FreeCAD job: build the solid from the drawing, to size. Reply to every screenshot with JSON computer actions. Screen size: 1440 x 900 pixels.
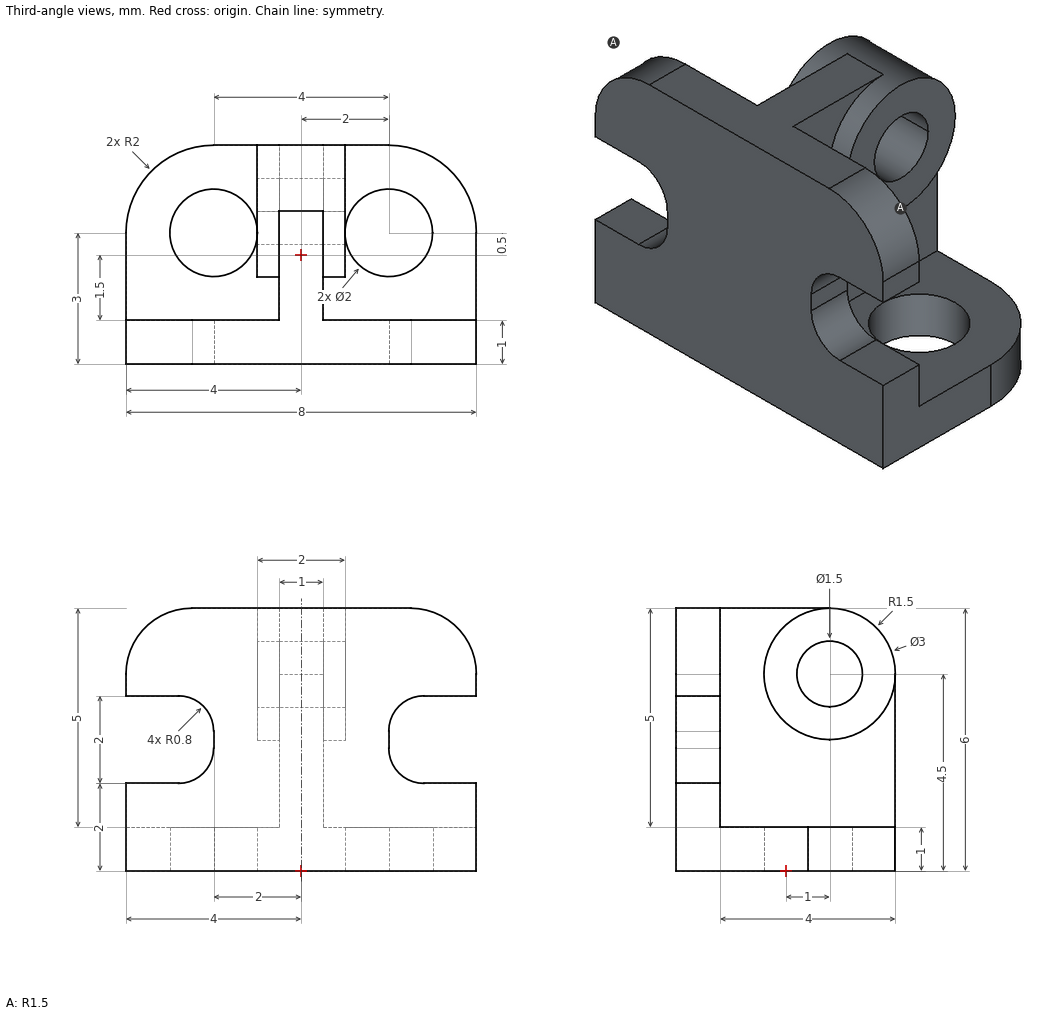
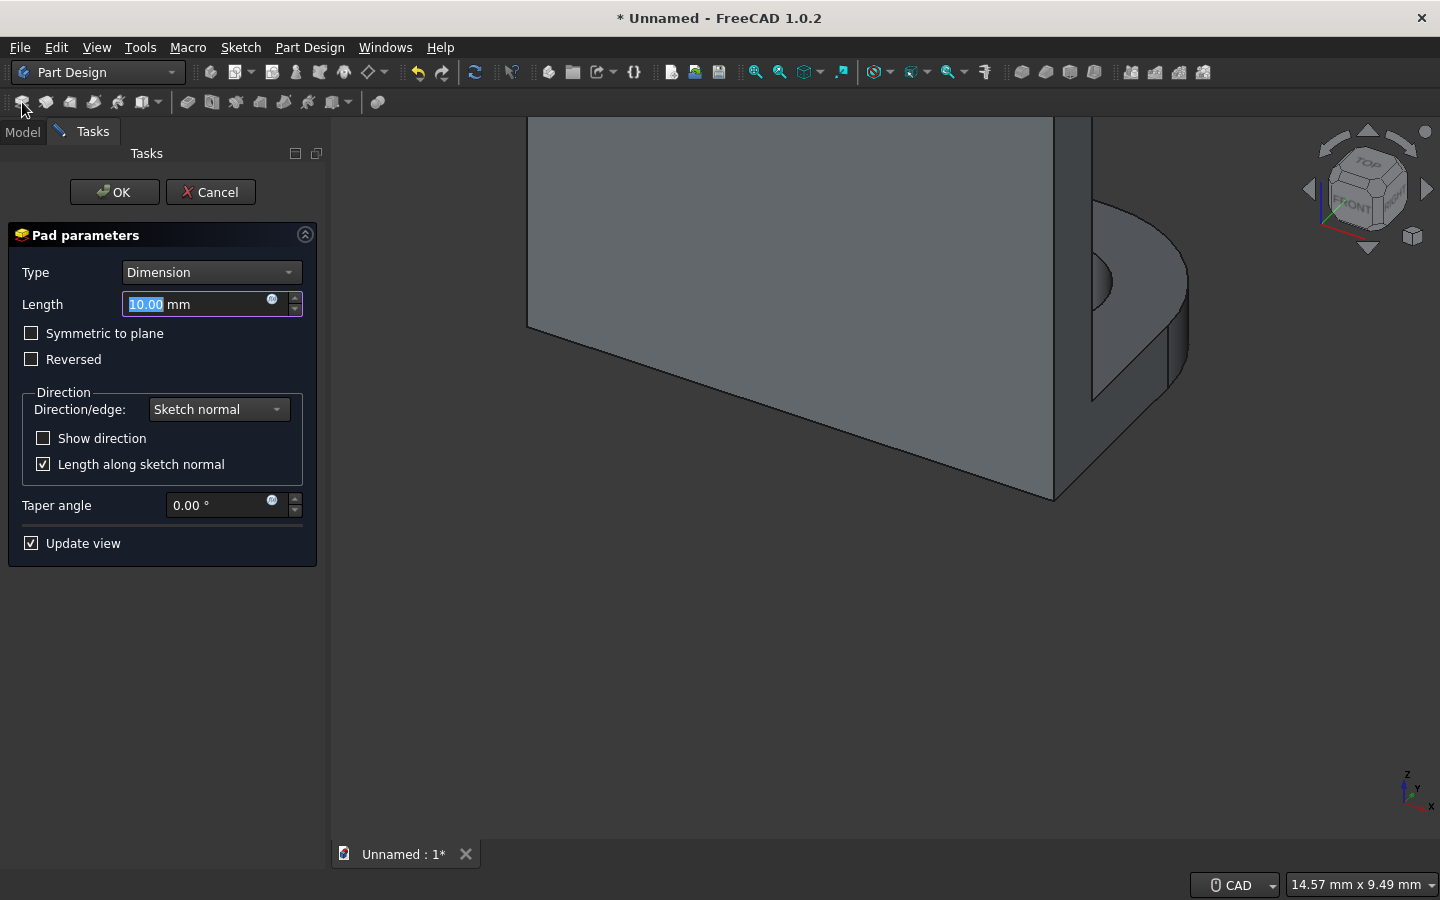
{"action": "type", "text": "5"}
{"action": "key", "text": "Tab"}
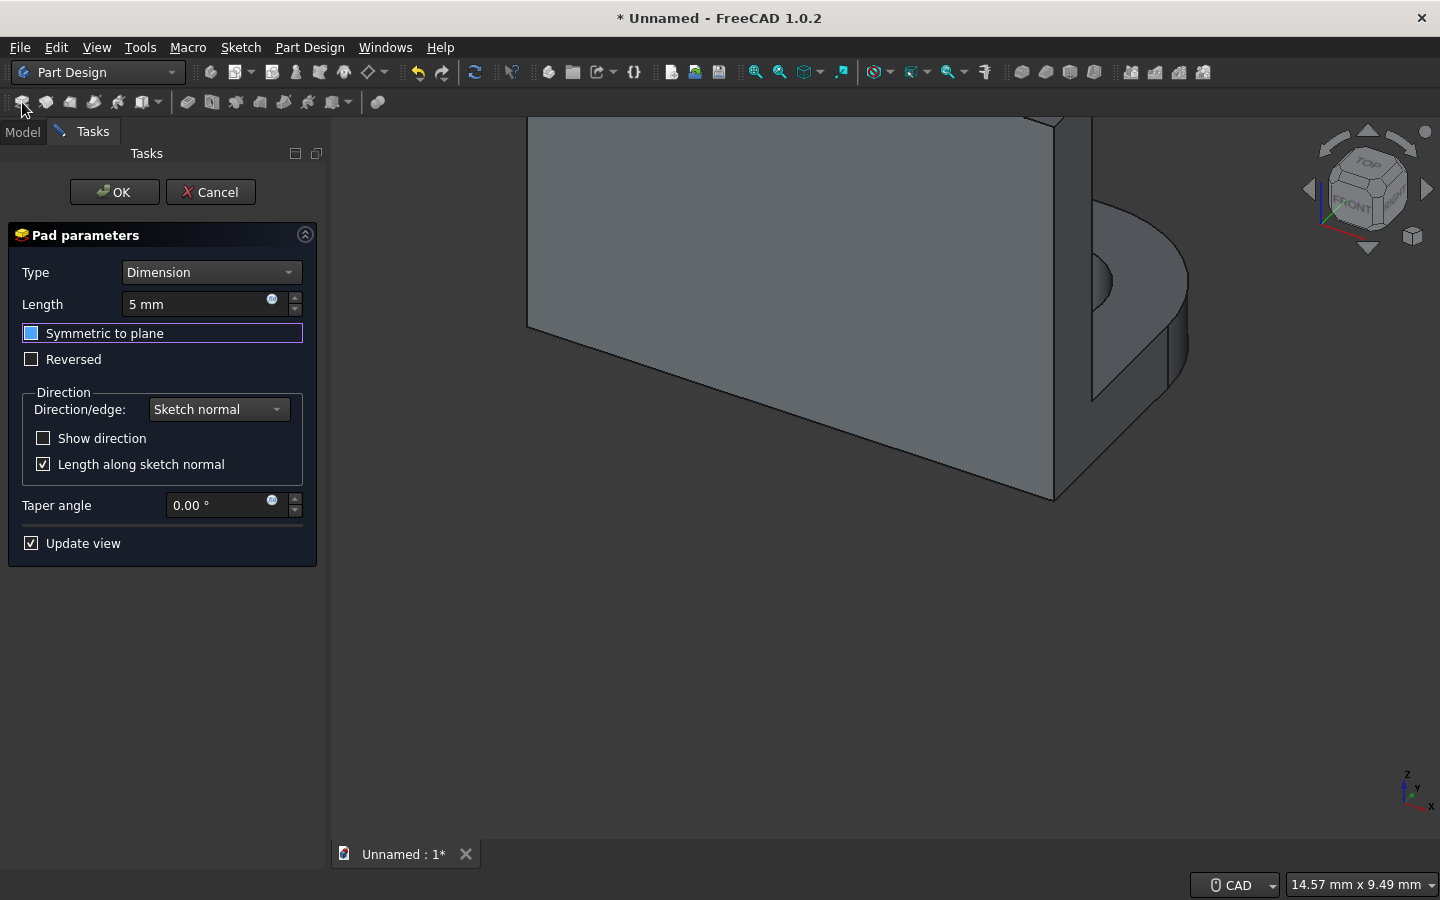
{"action": "left_click", "coordinate": [115, 192]}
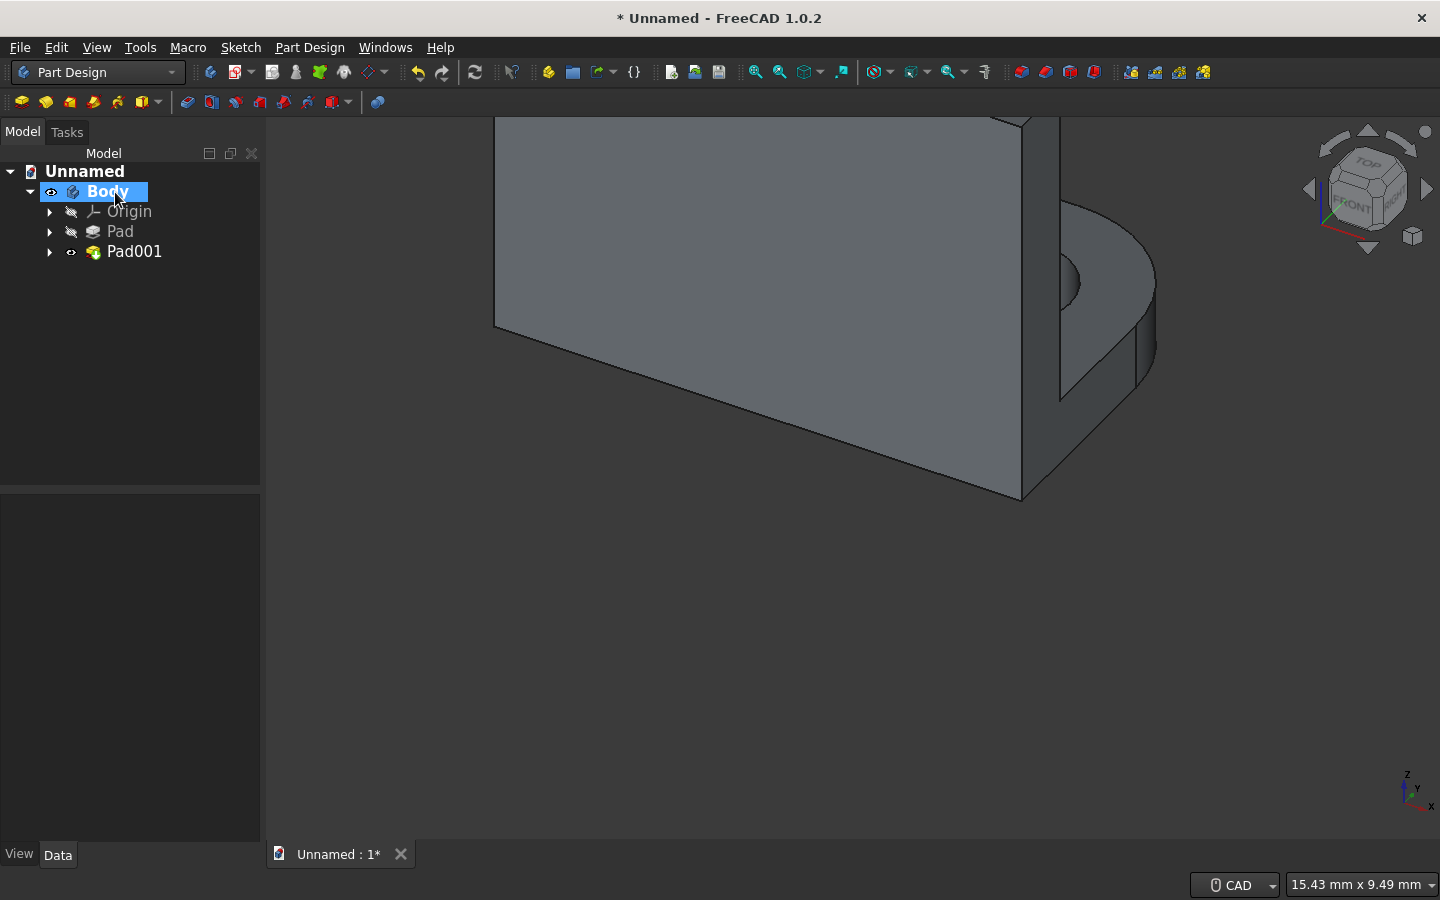
{"action": "left_click", "coordinate": [756, 72]}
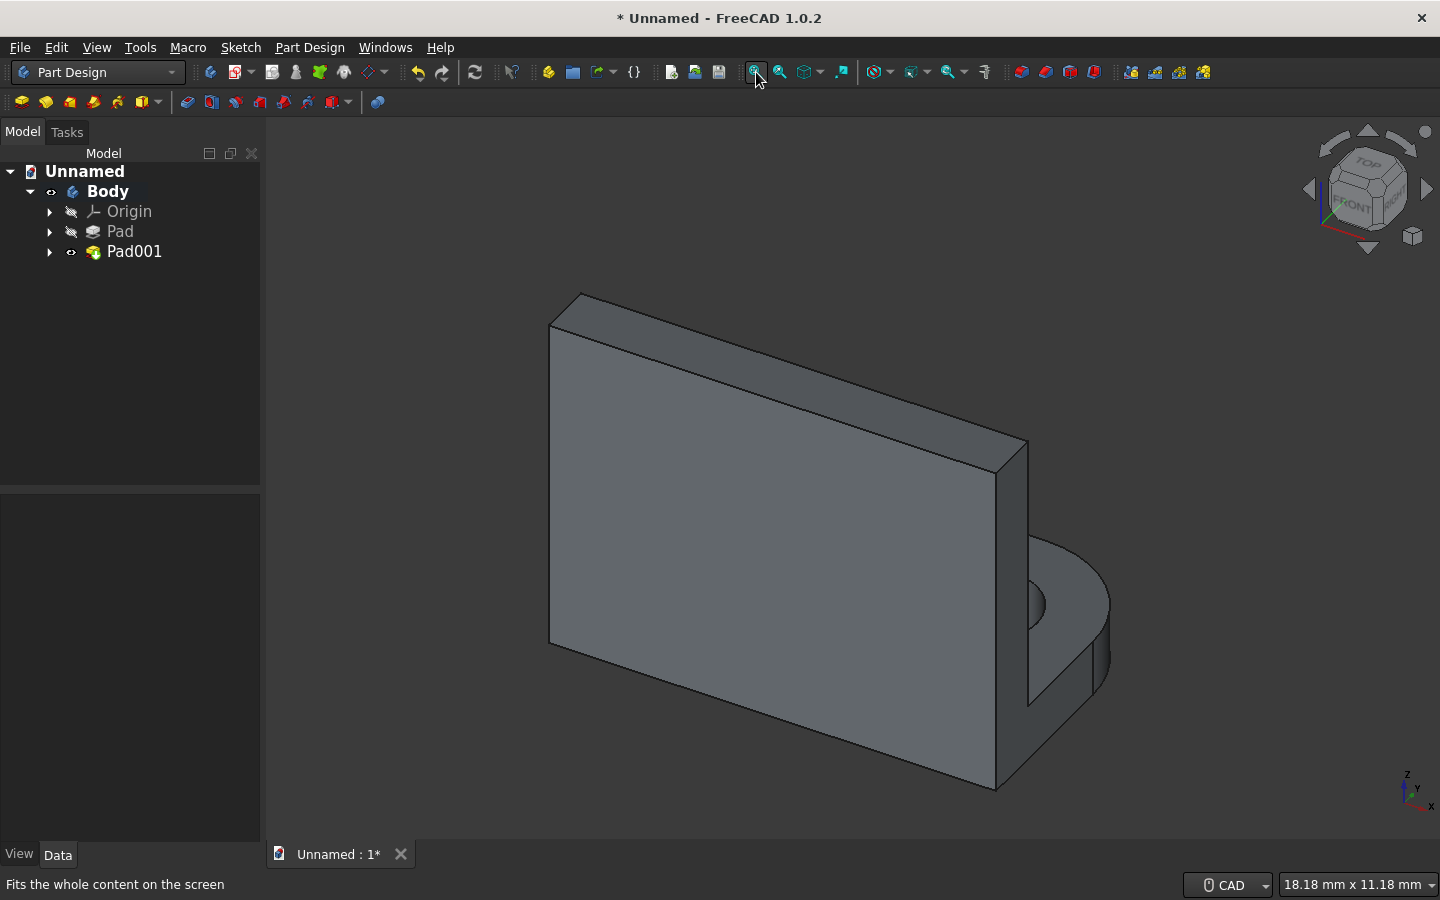
{"action": "key", "text": "4"}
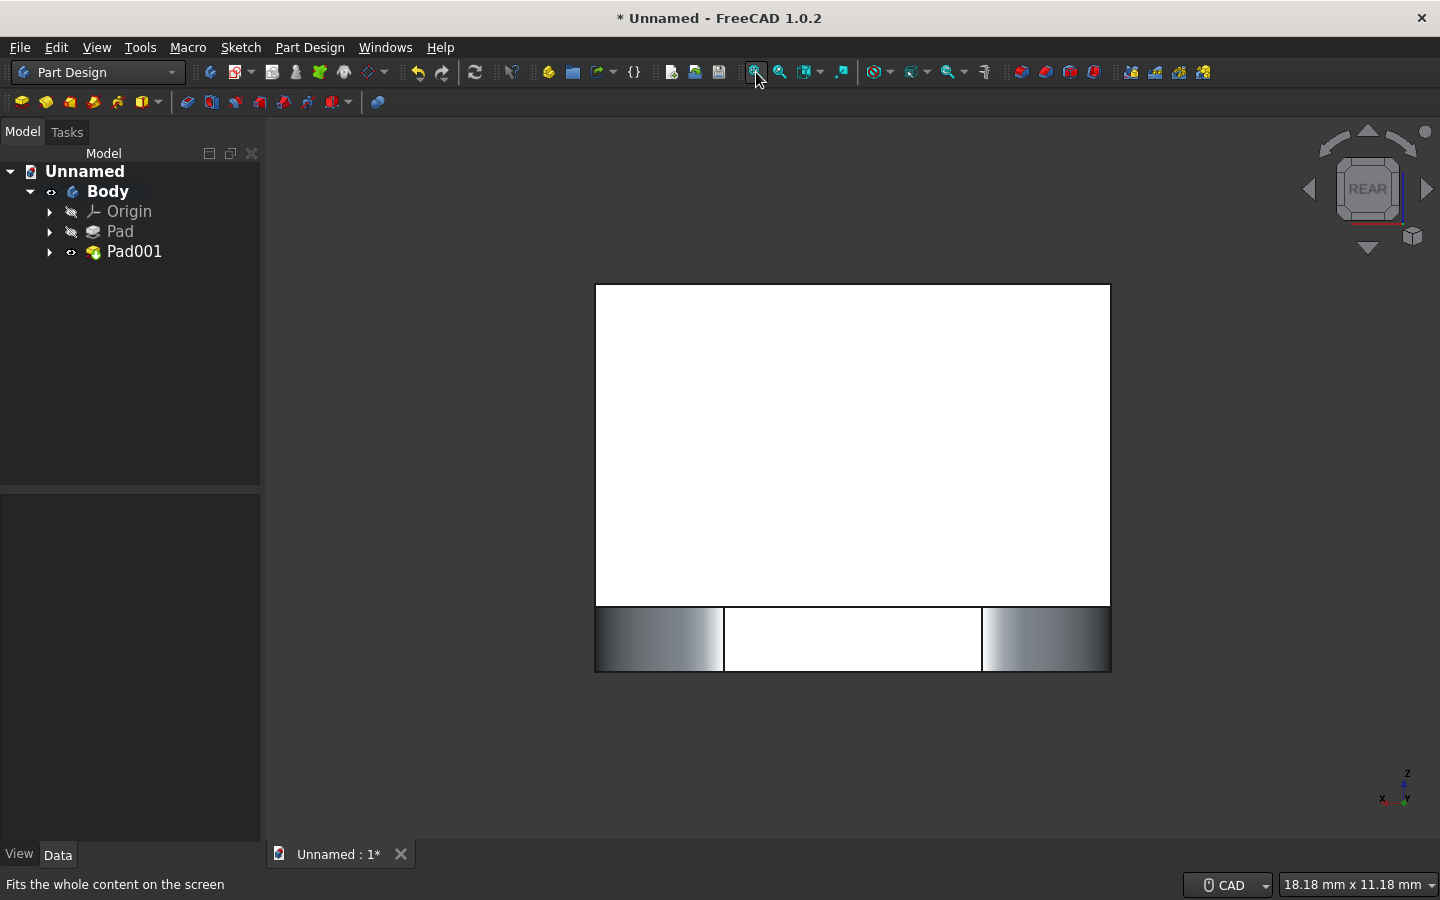
{"action": "left_click", "coordinate": [779, 445]}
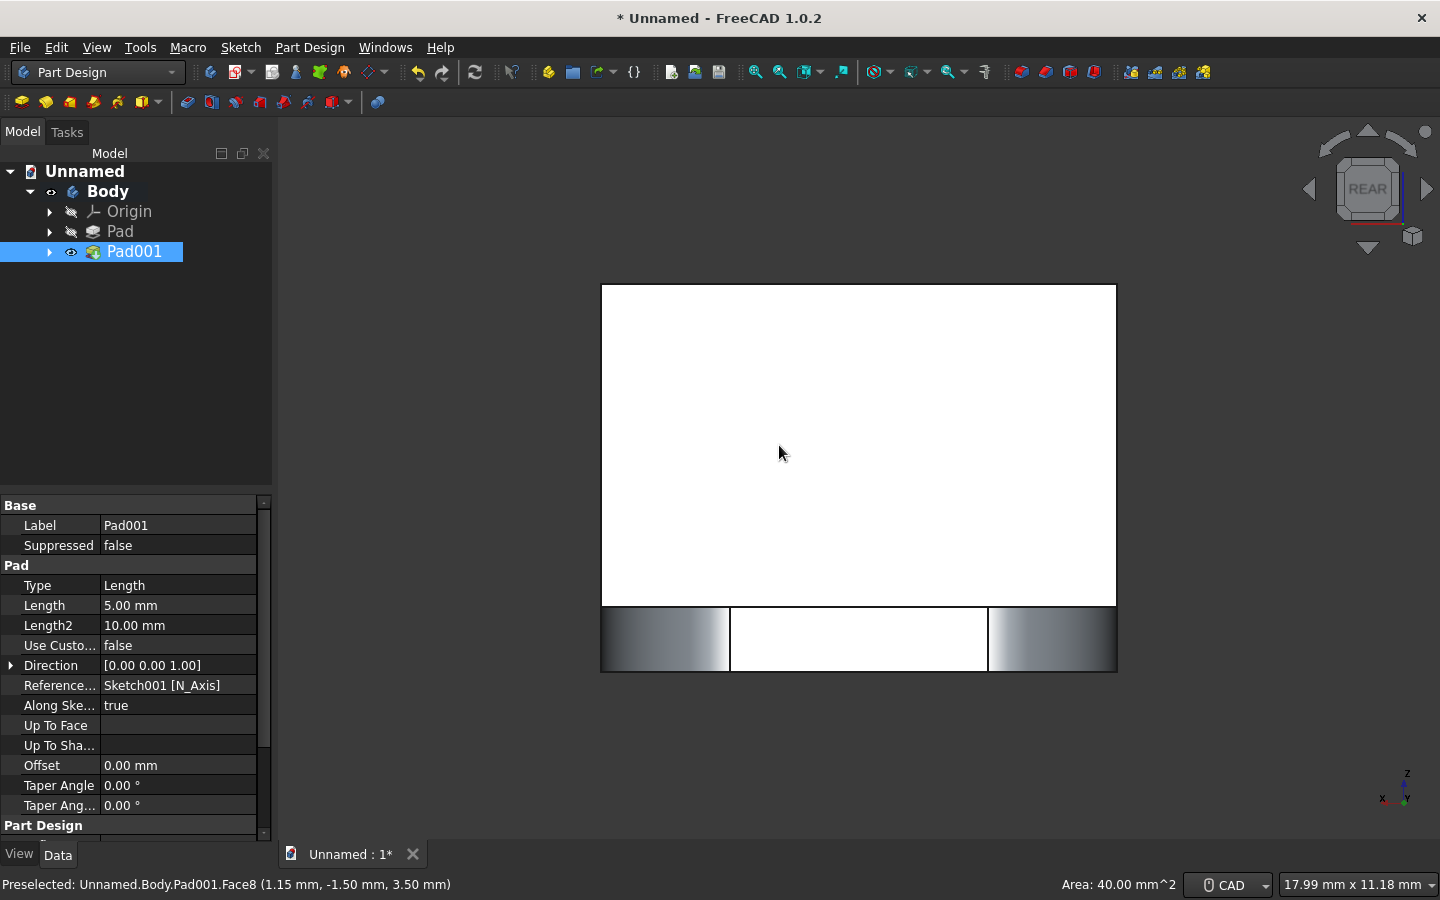
{"action": "left_click", "coordinate": [236, 72]}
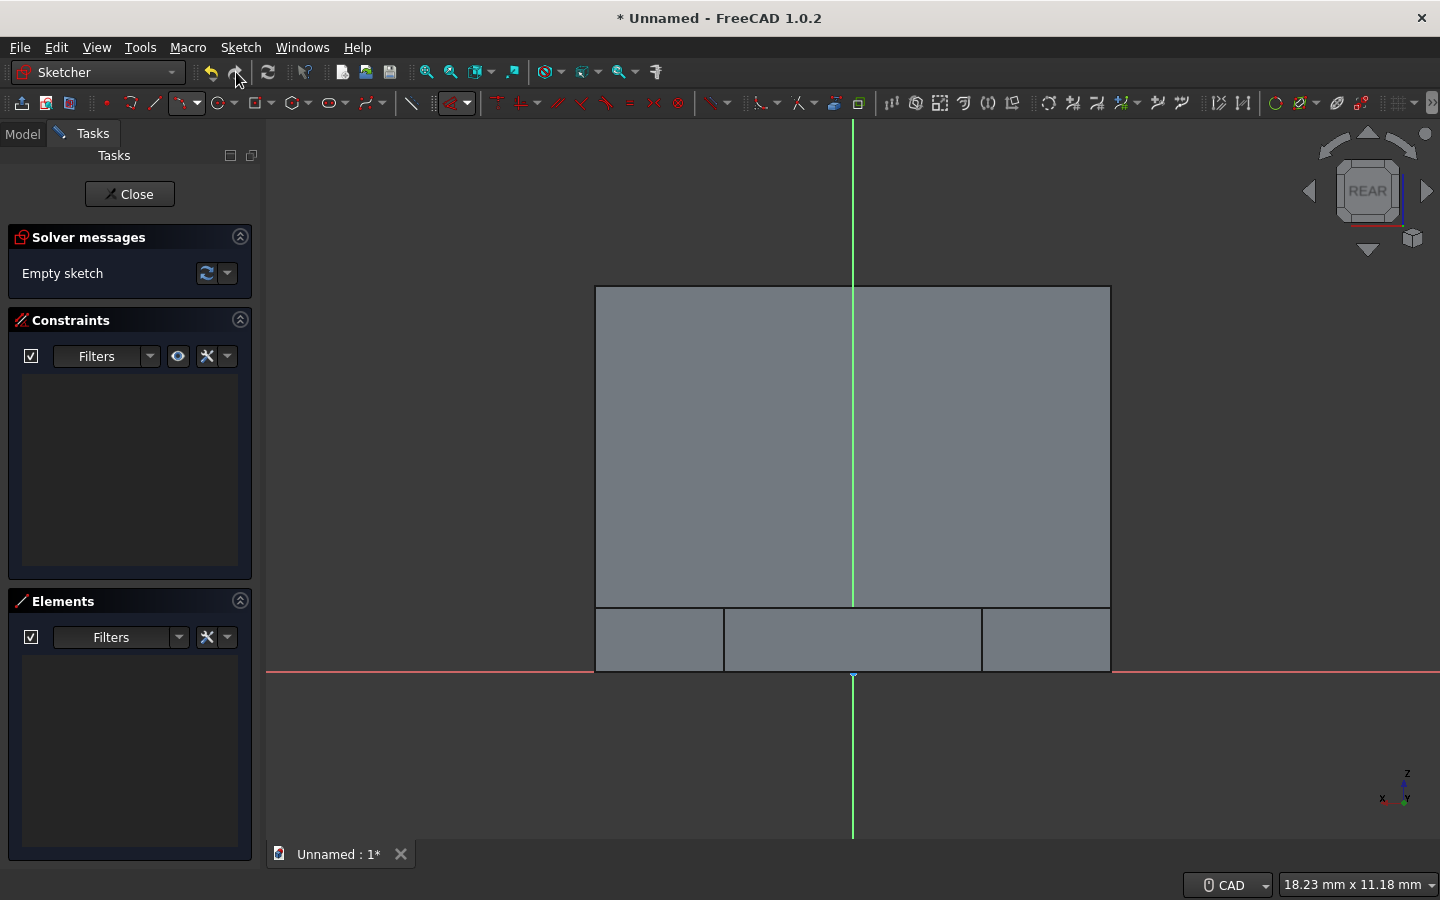
{"action": "left_click", "coordinate": [70, 104]}